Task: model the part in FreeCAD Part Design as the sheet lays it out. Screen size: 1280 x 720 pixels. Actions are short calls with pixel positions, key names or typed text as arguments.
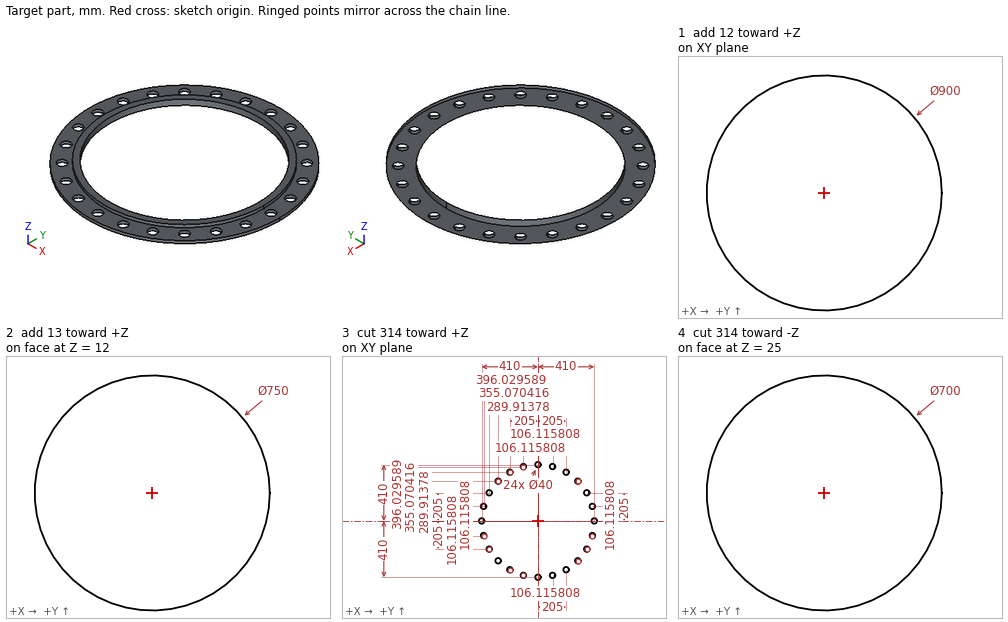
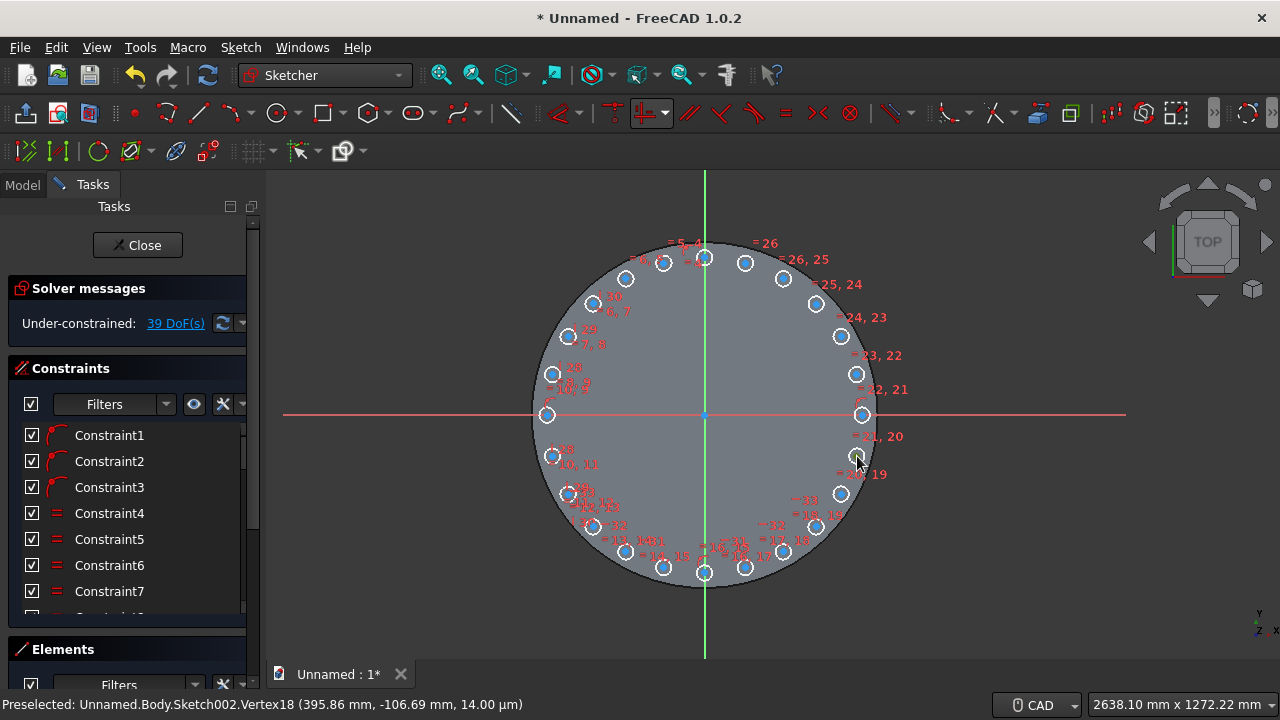
click(857, 375)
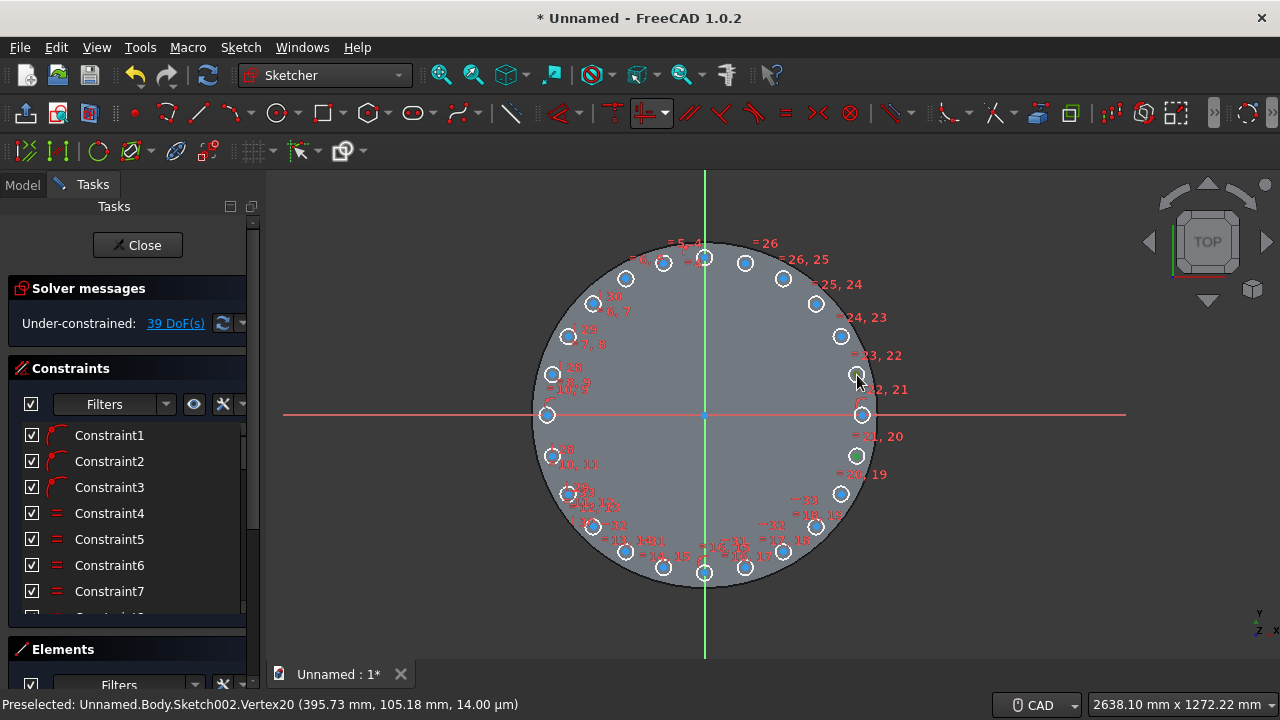
key(v)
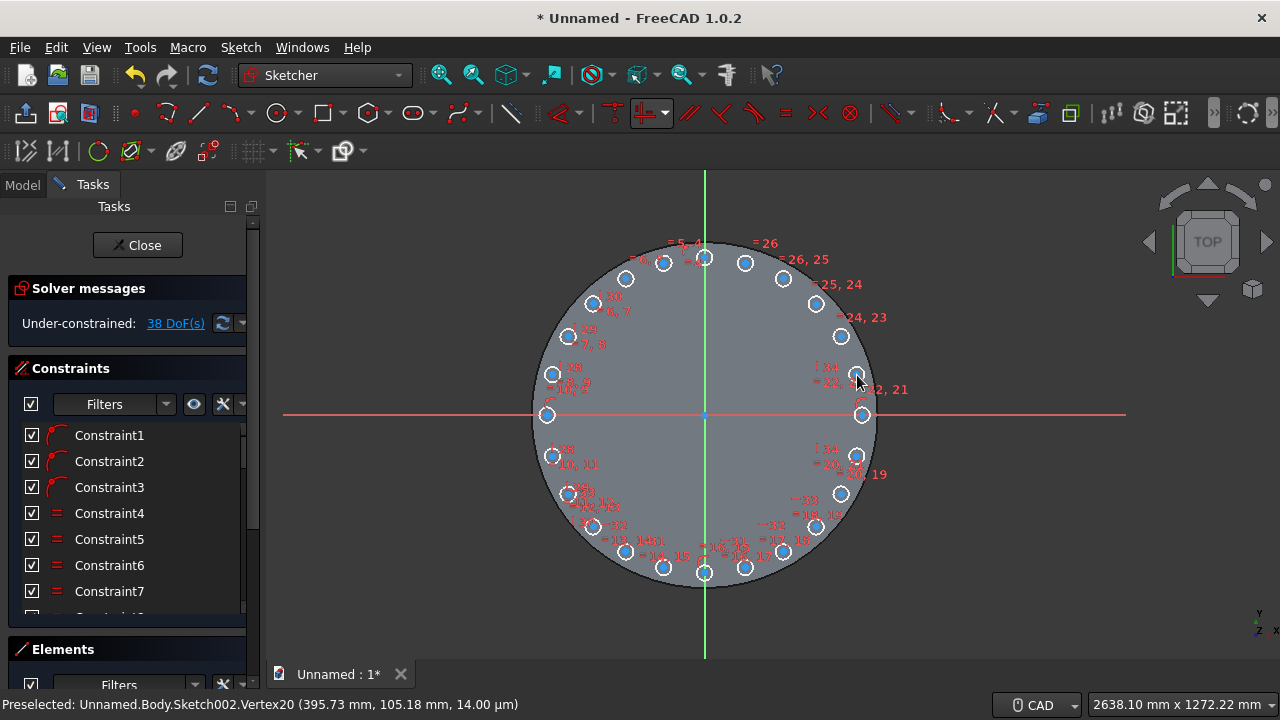
click(843, 496)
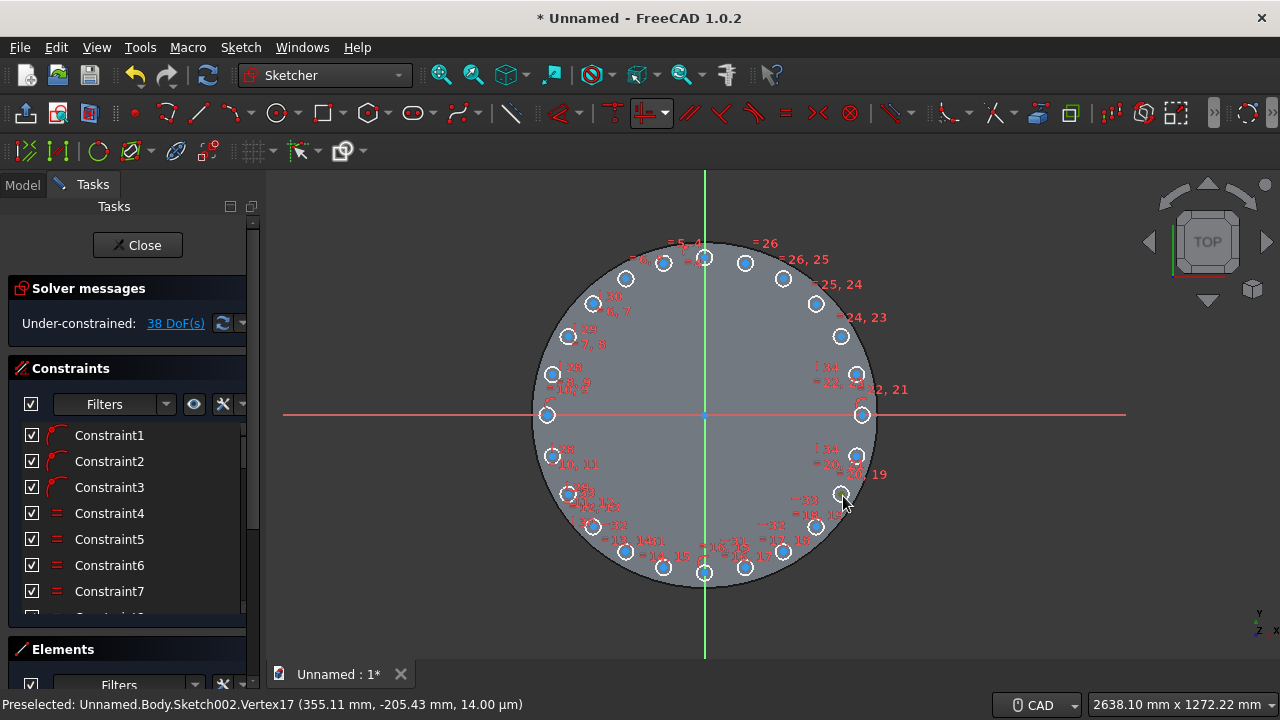
click(841, 337)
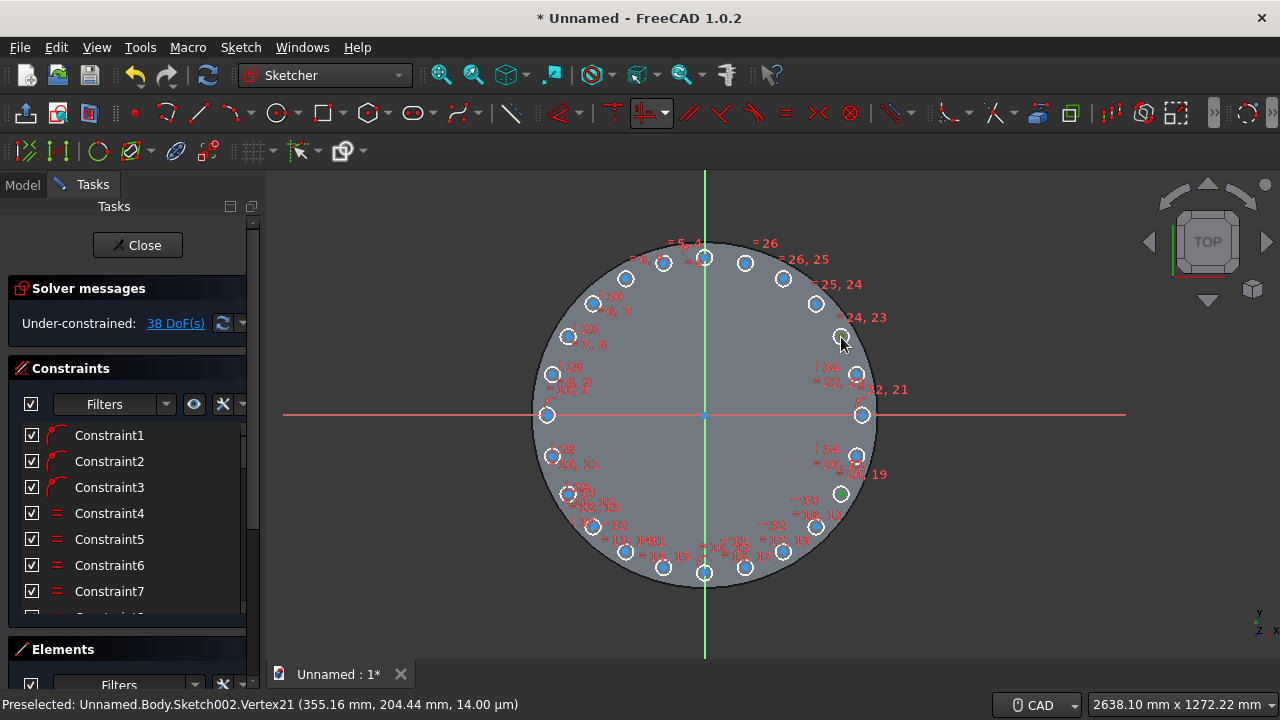
key(v)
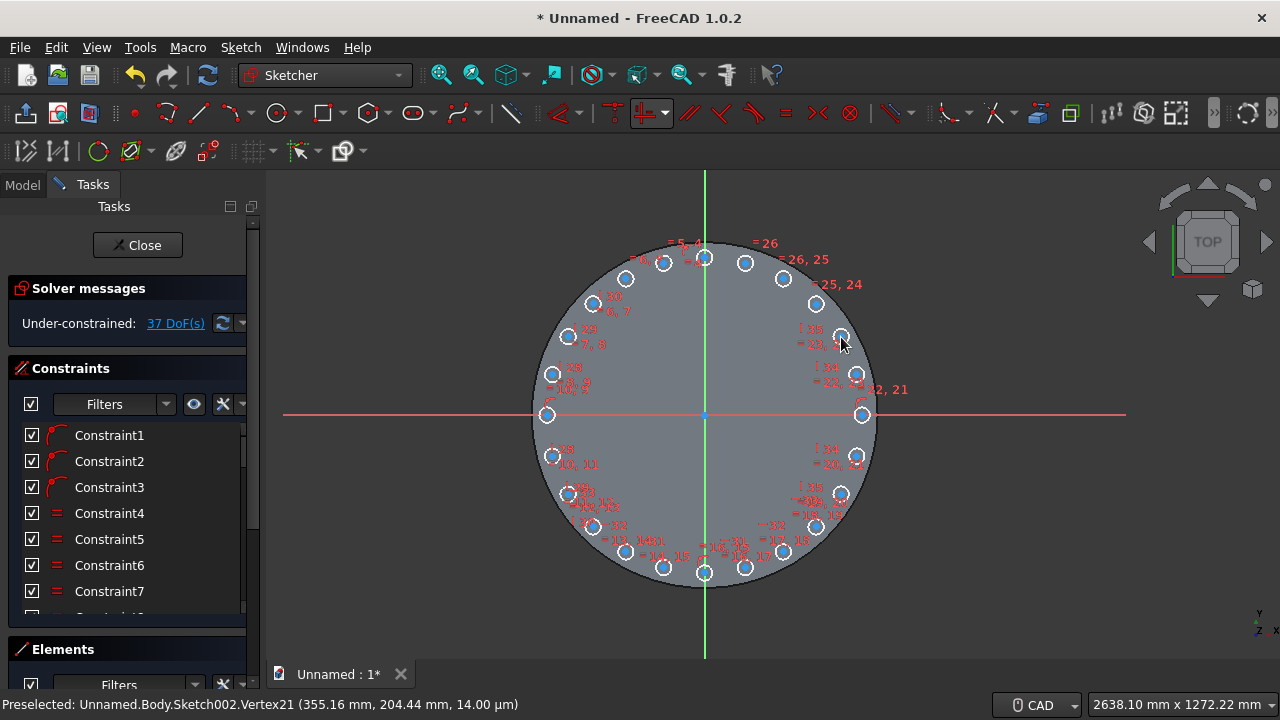
click(626, 279)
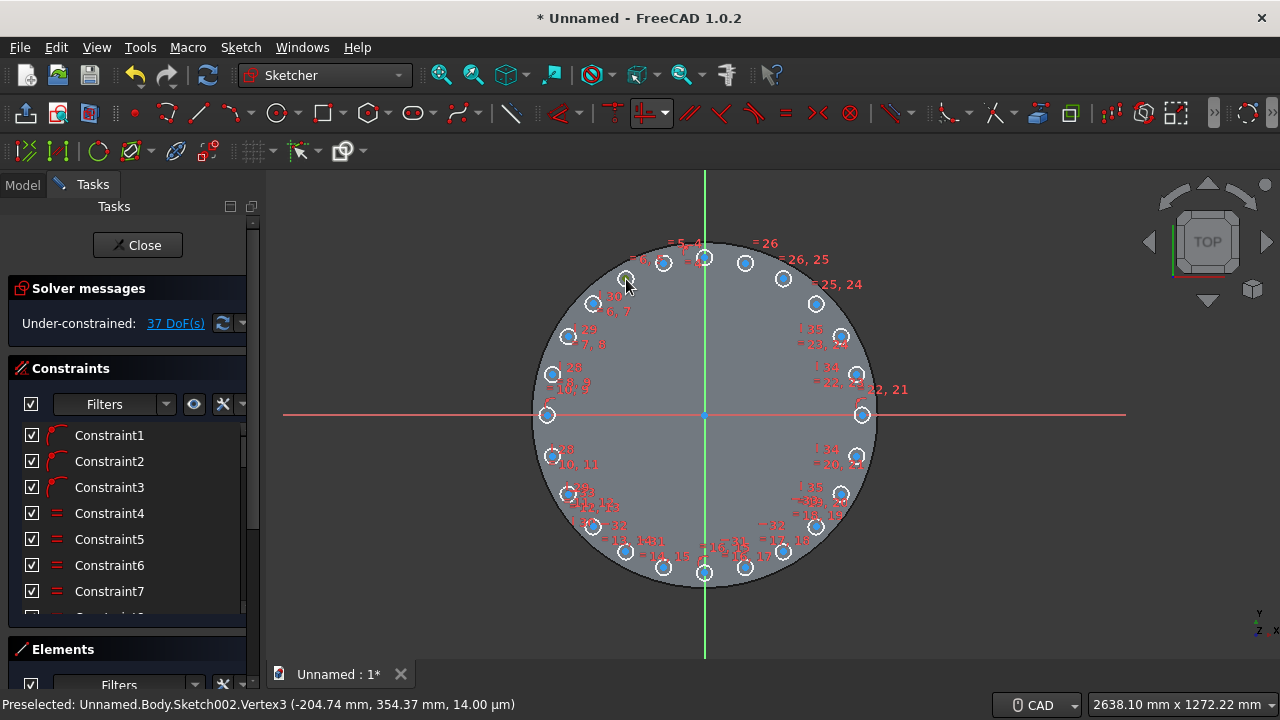
click(783, 279)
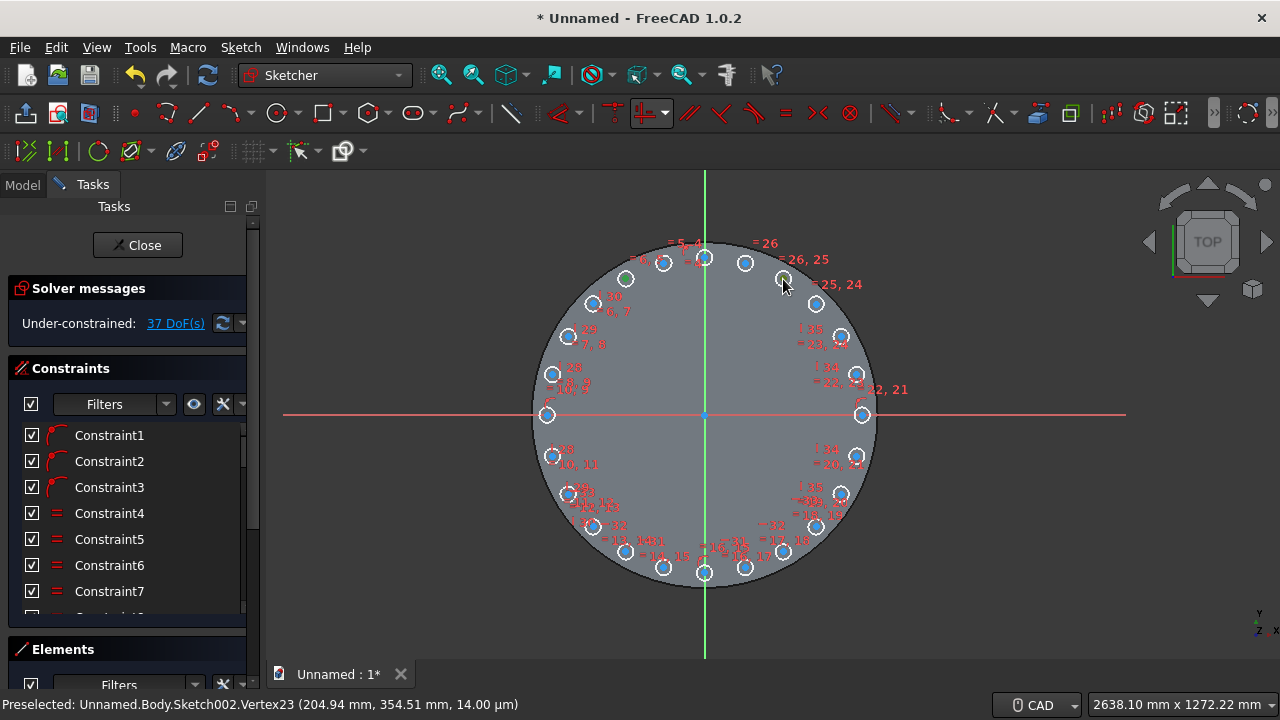
click(668, 114)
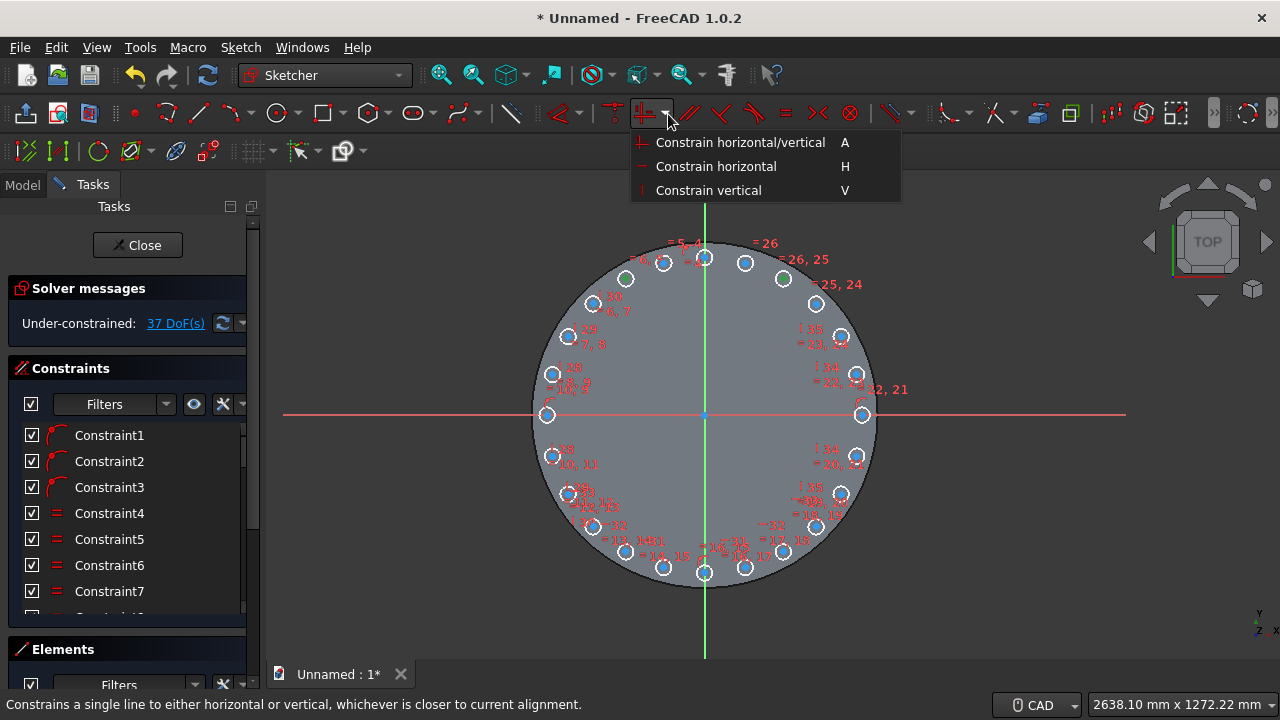
click(766, 166)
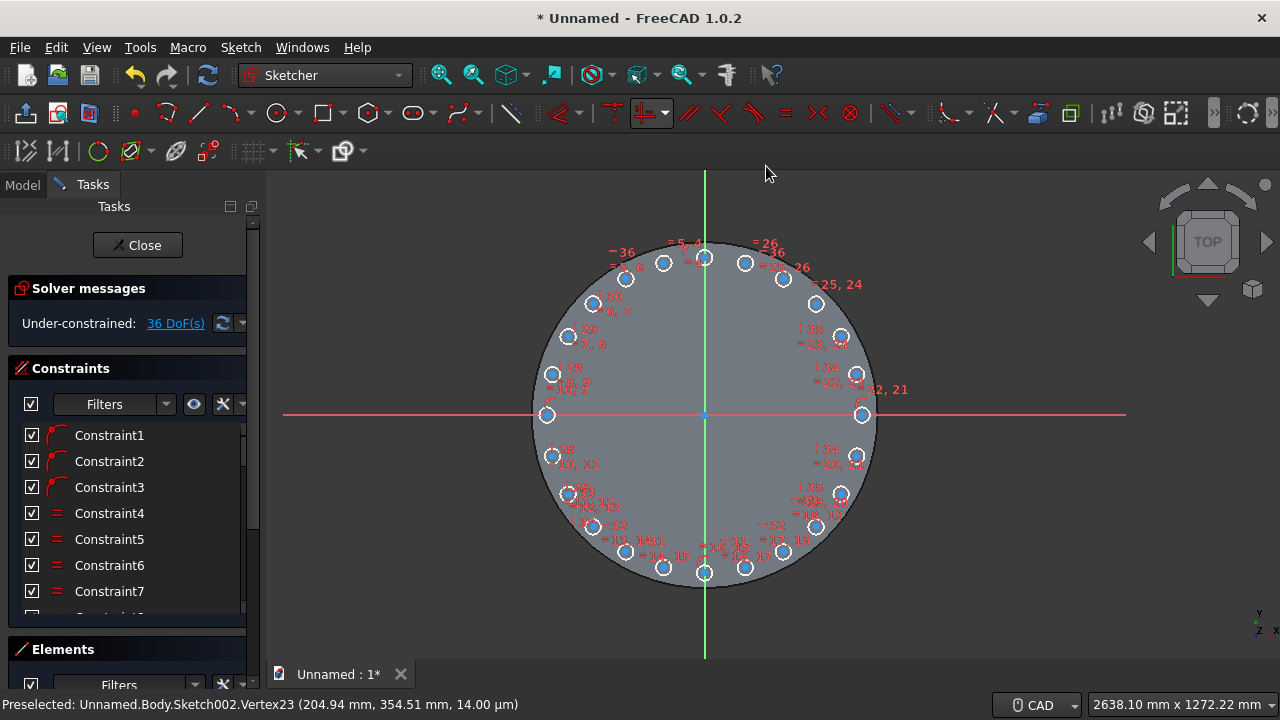
click(664, 263)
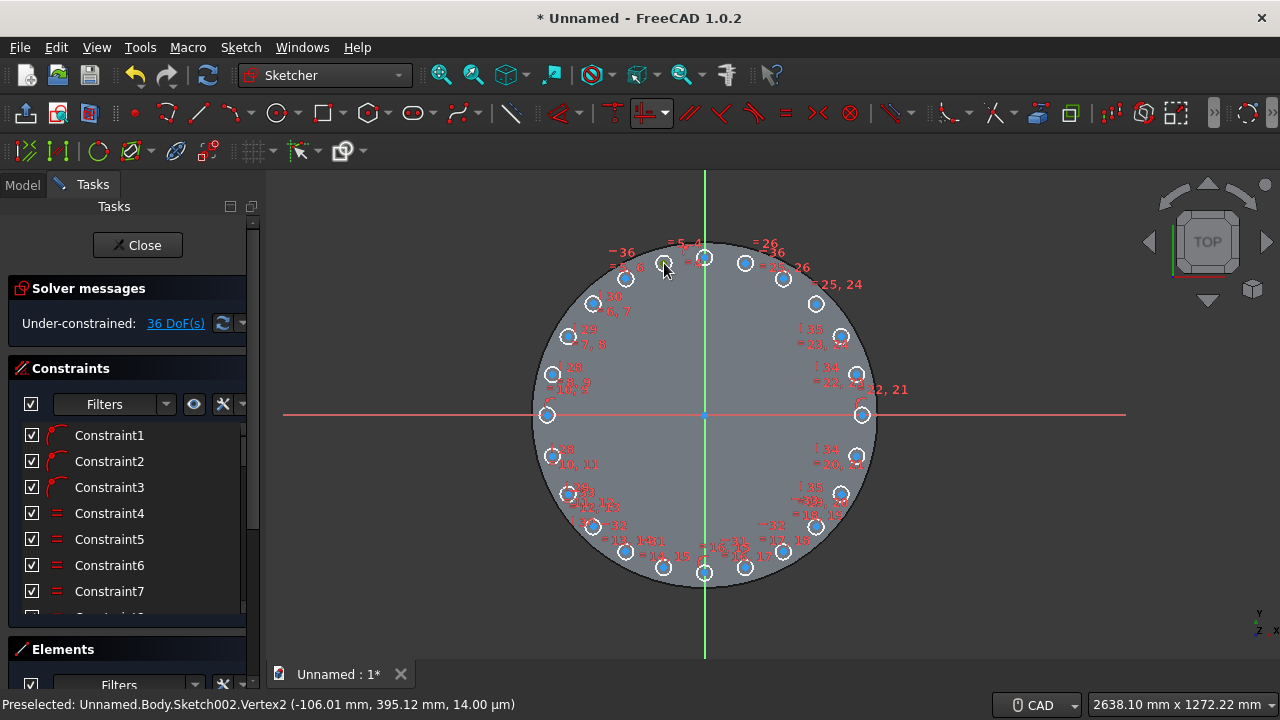
click(745, 263)